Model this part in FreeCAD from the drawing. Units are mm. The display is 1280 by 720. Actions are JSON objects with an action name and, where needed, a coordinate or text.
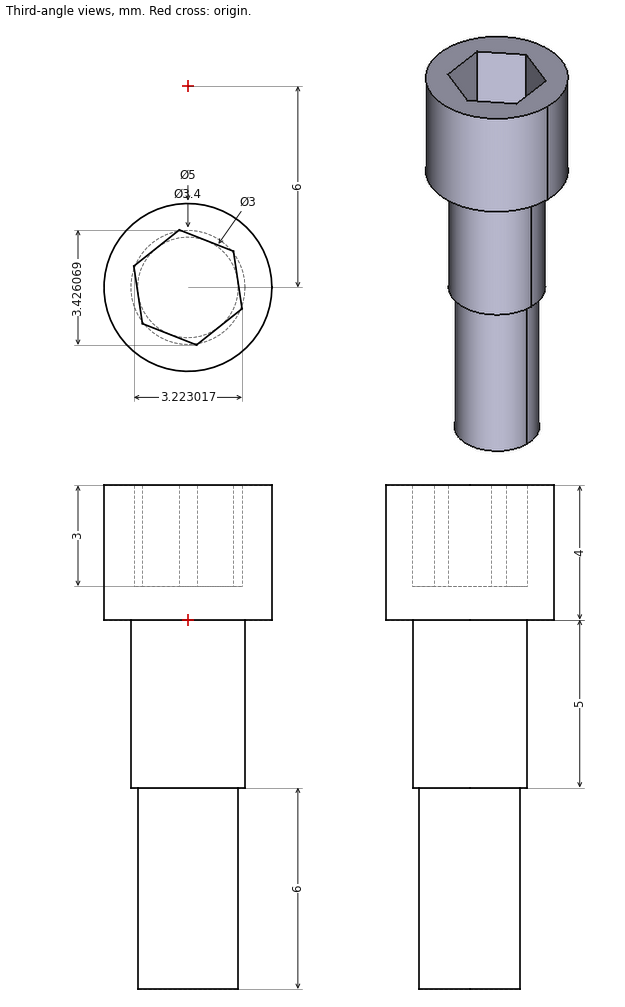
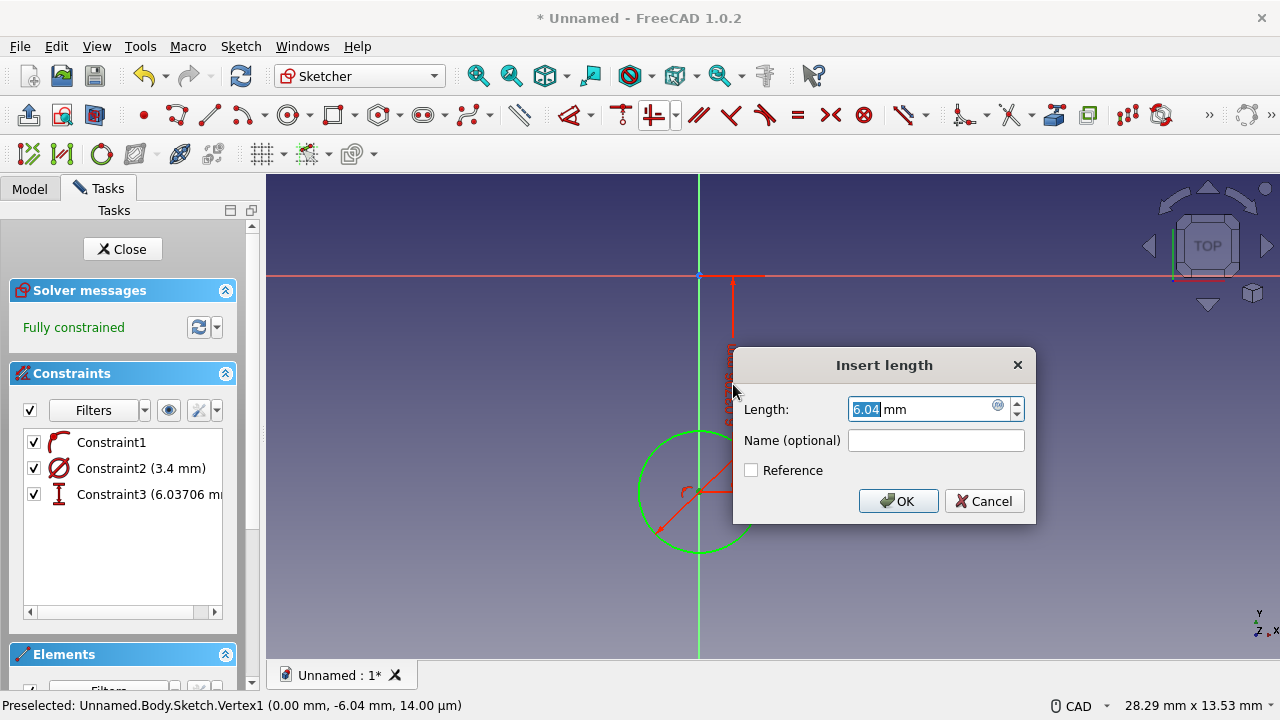
{"action": "type", "text": "6"}
{"action": "key", "text": "Return"}
{"action": "key", "text": "Escape"}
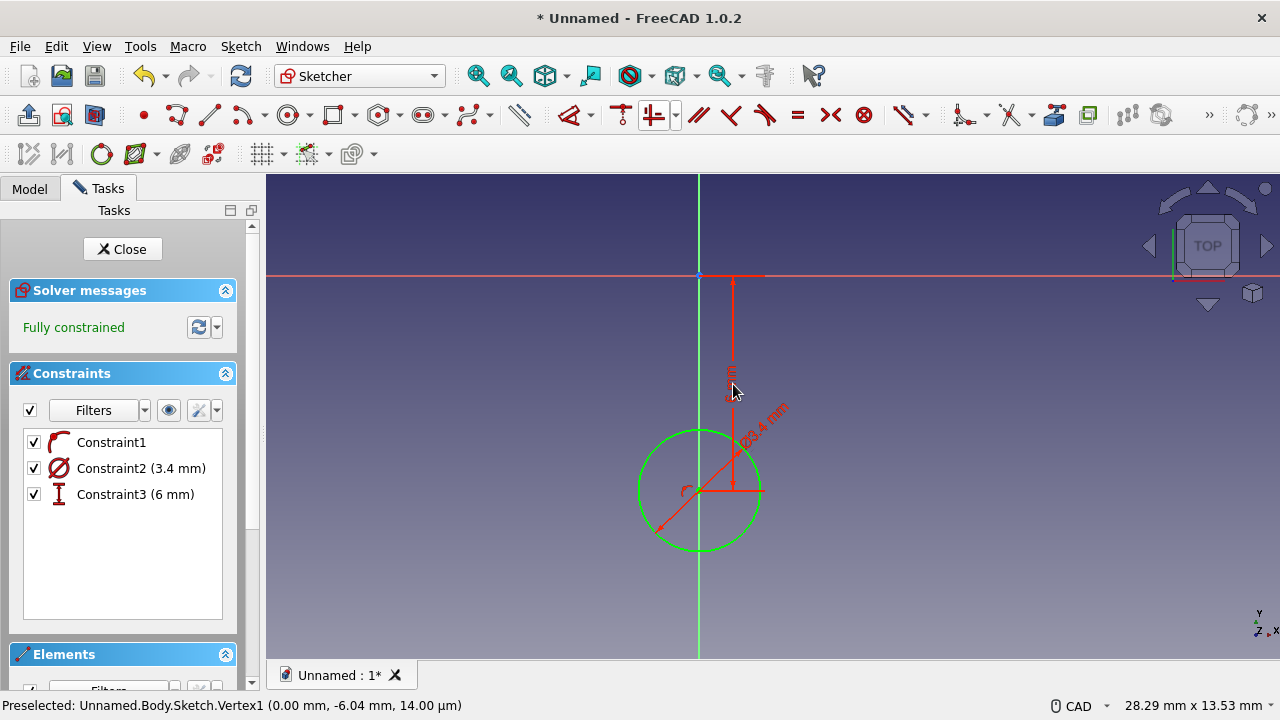
{"action": "left_click", "coordinate": [123, 249]}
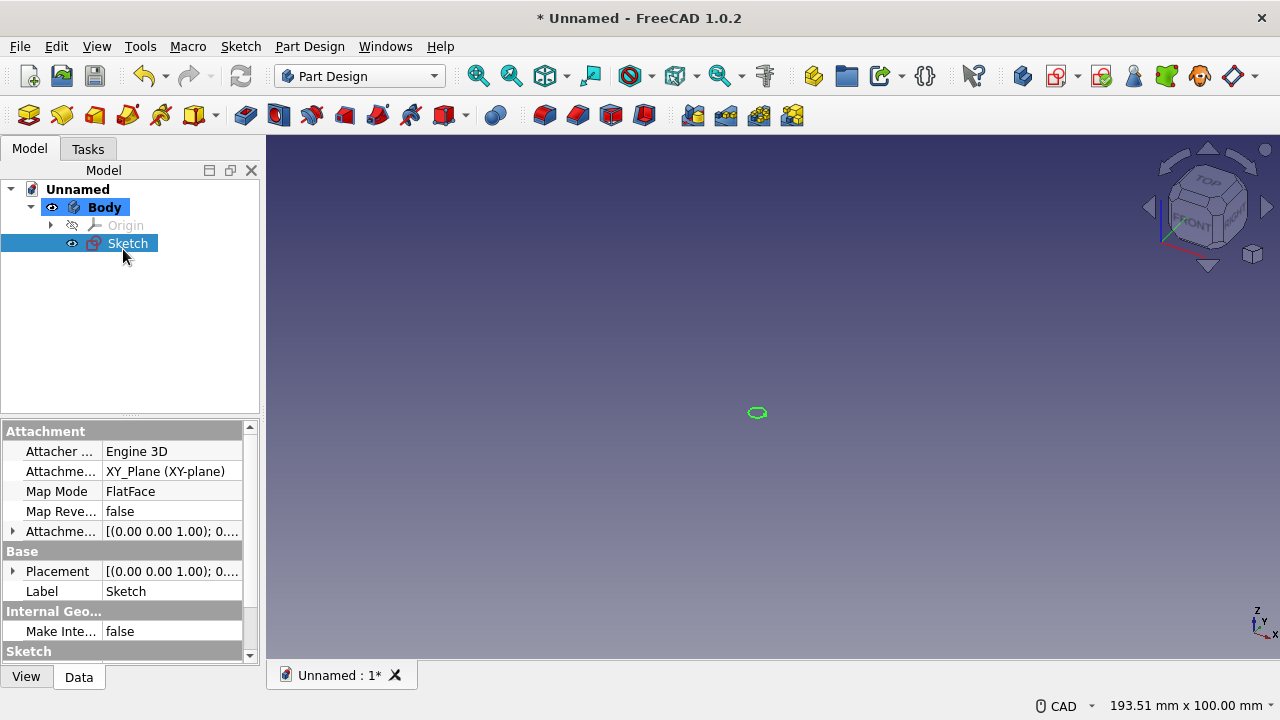
{"action": "left_click", "coordinate": [29, 116]}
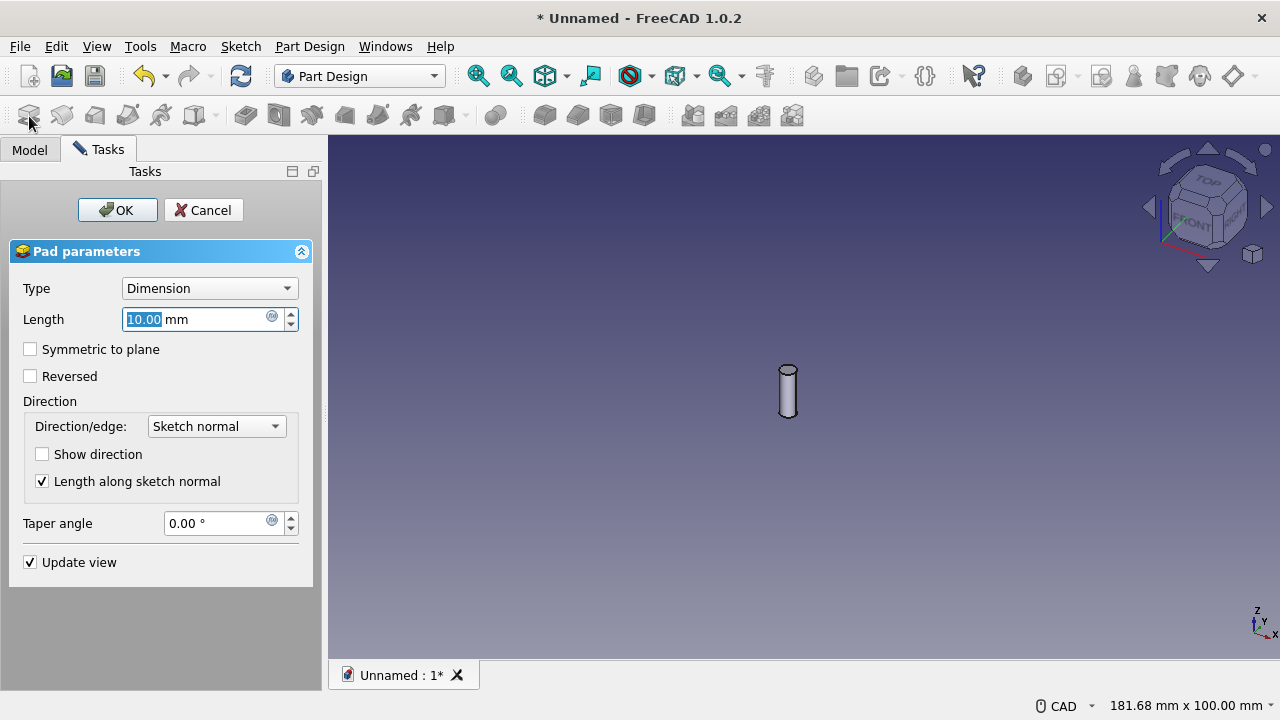
{"action": "type", "text": "5"}
{"action": "key", "text": "Tab"}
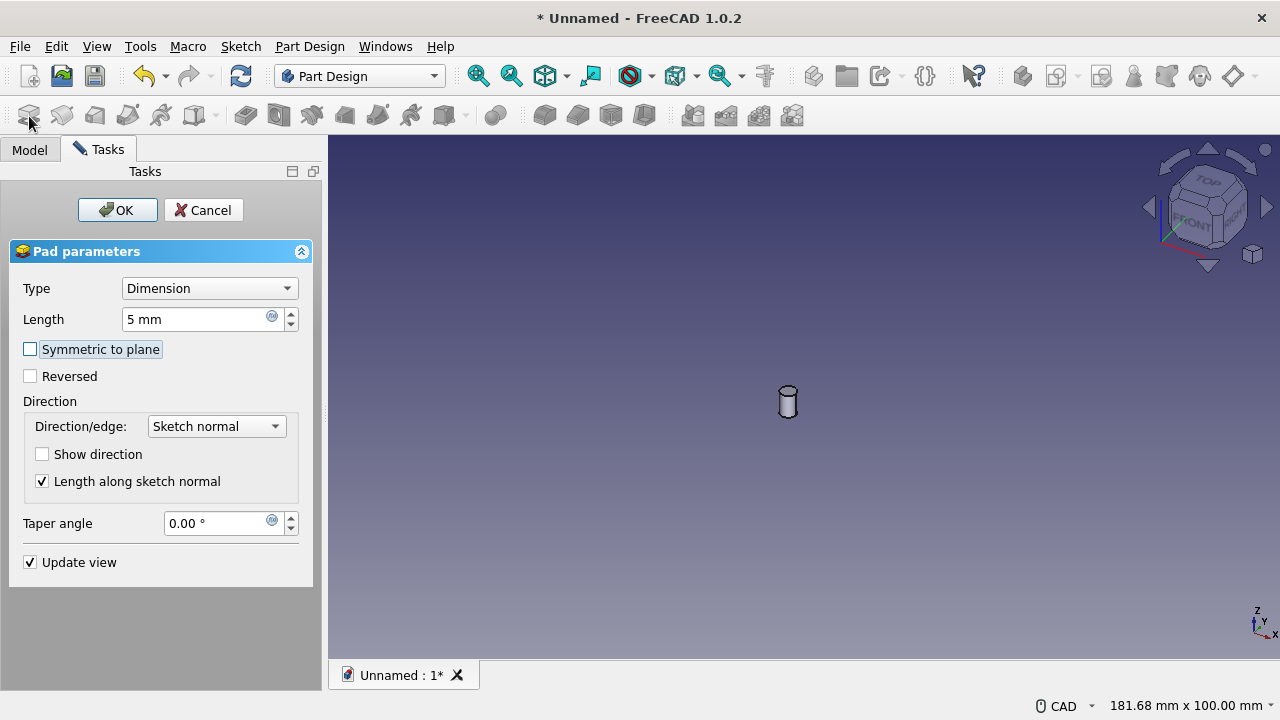
{"action": "left_click", "coordinate": [31, 376]}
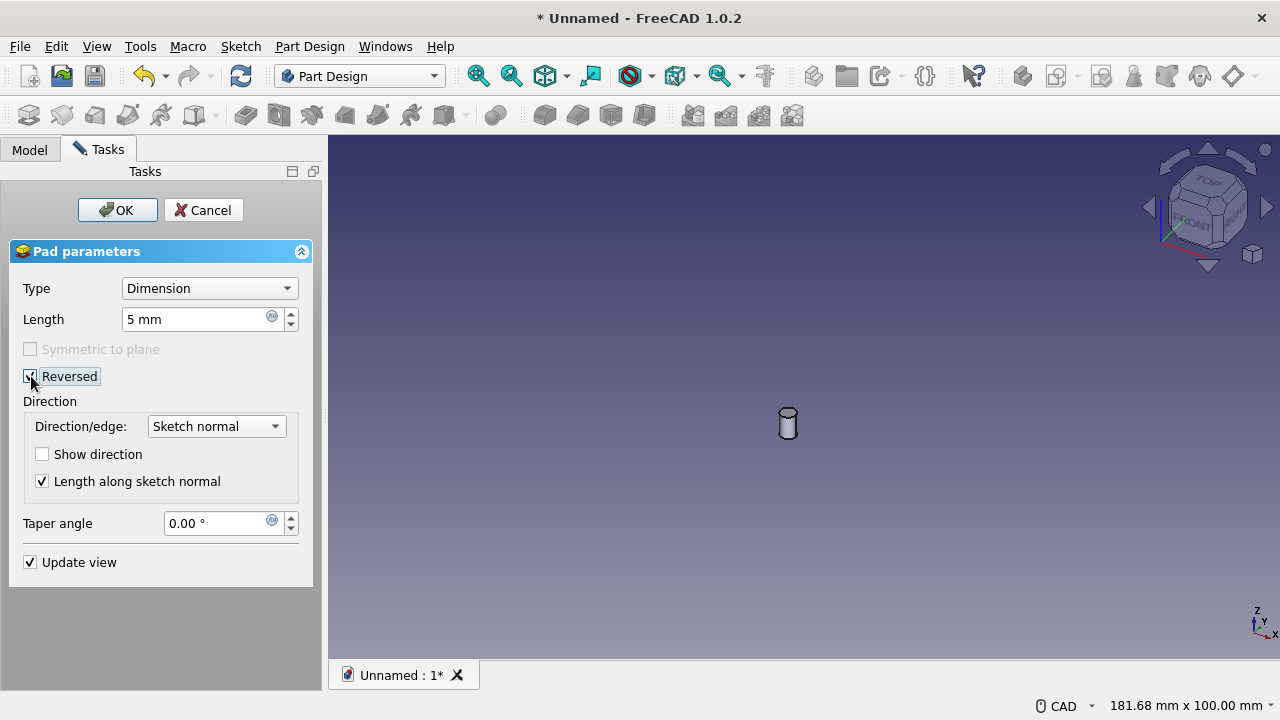
{"action": "left_click", "coordinate": [118, 210]}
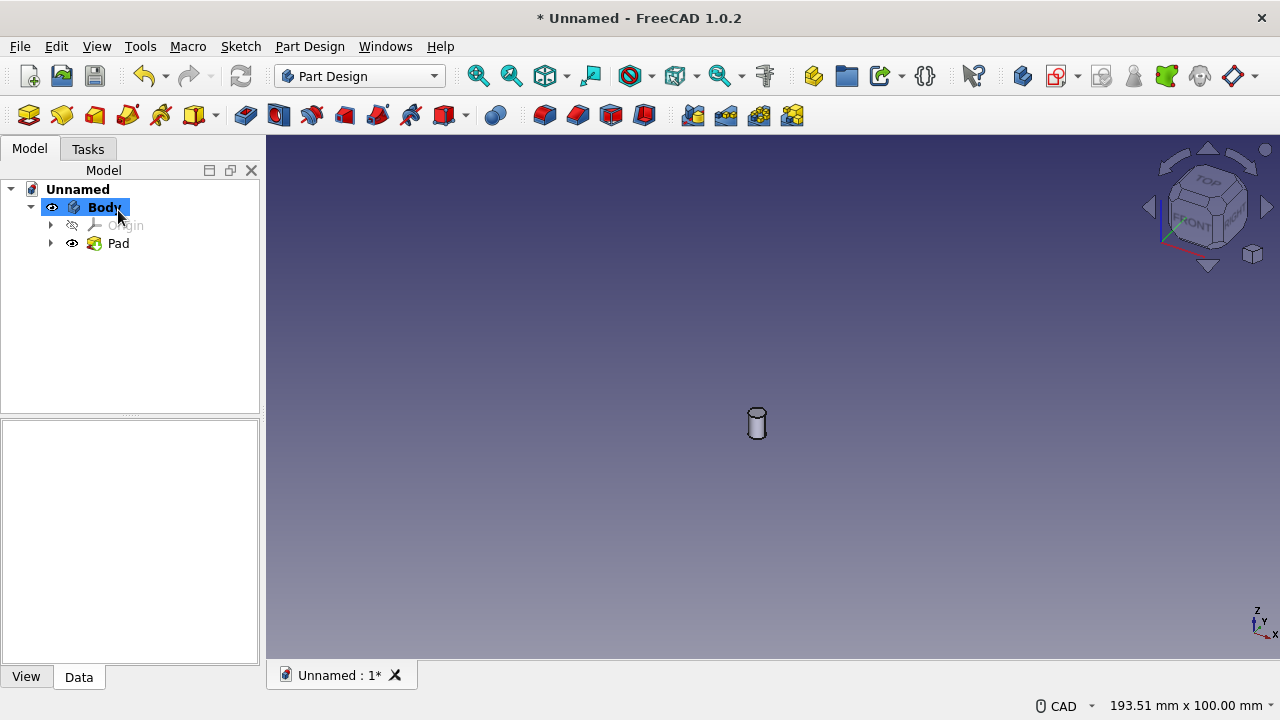
{"action": "left_click", "coordinate": [479, 76]}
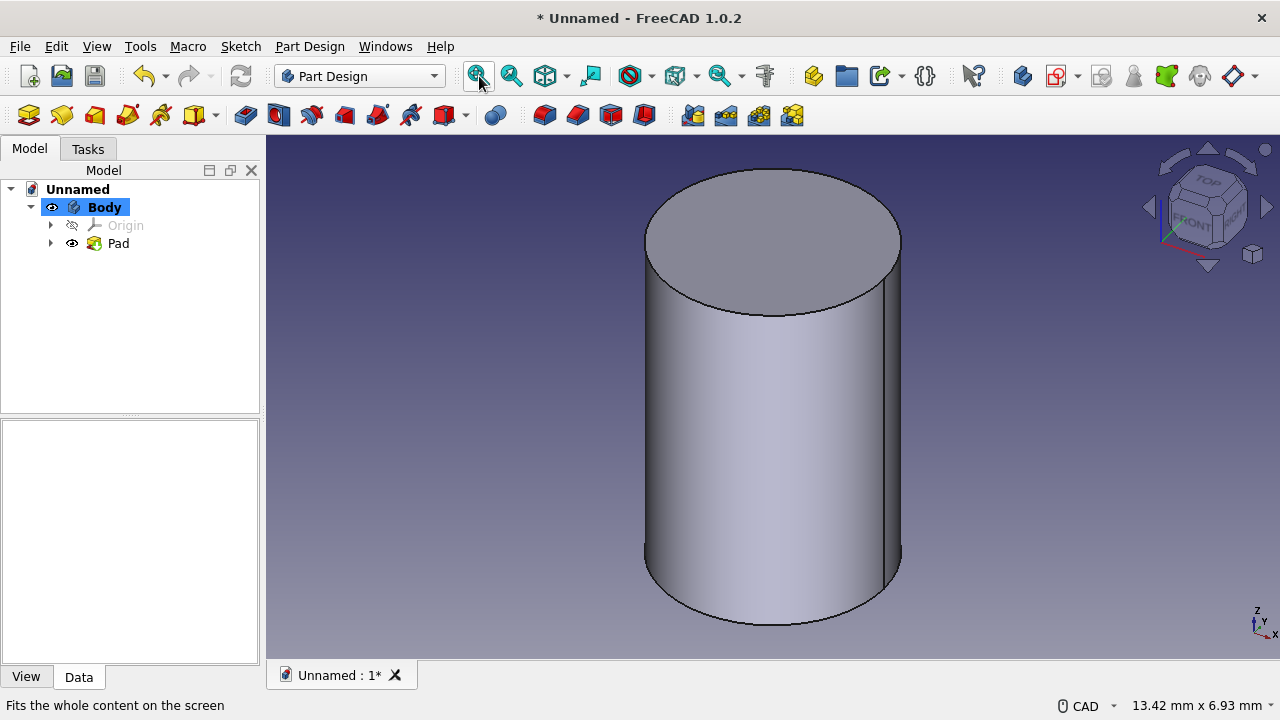
{"action": "key", "text": "5"}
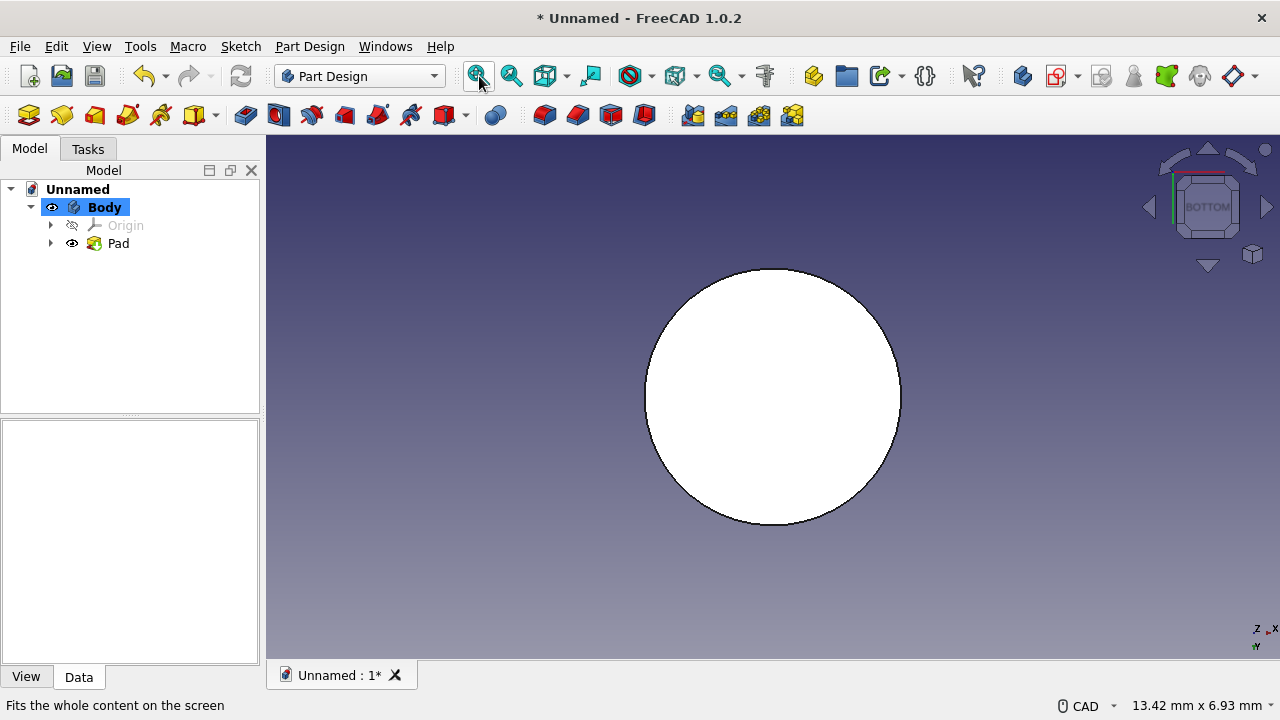
{"action": "left_click", "coordinate": [773, 396]}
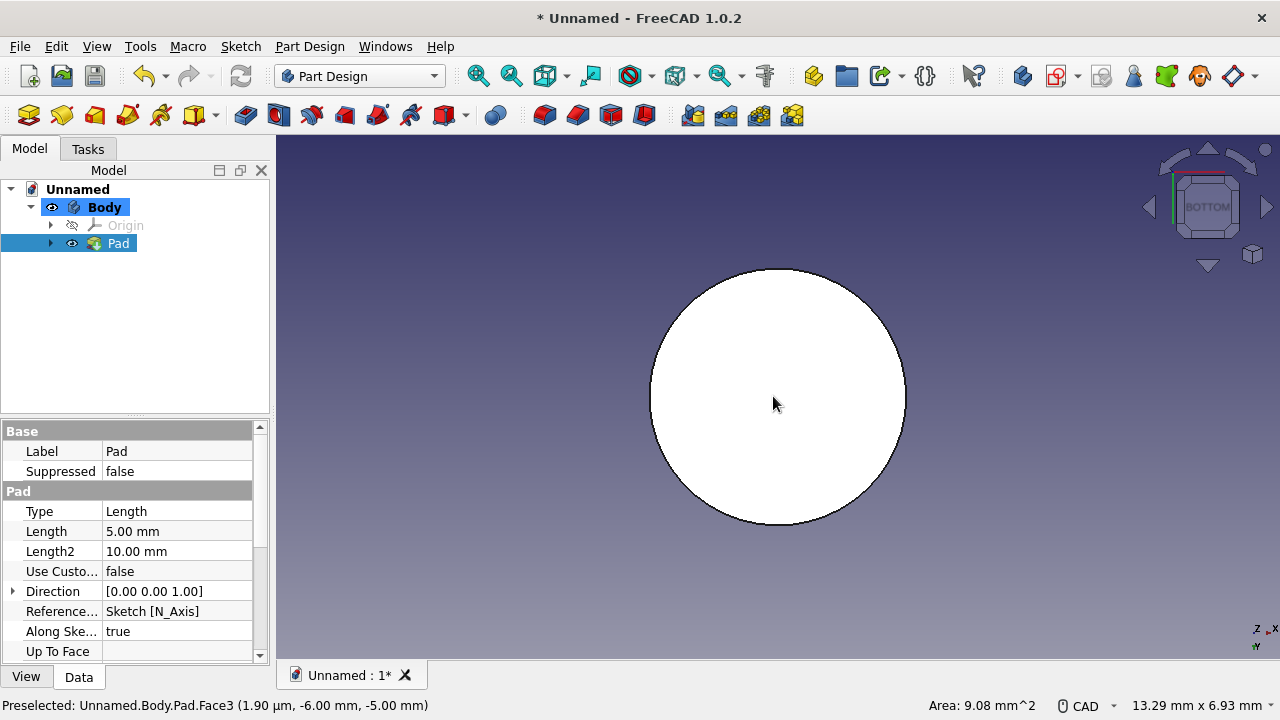
{"action": "left_click", "coordinate": [1056, 76]}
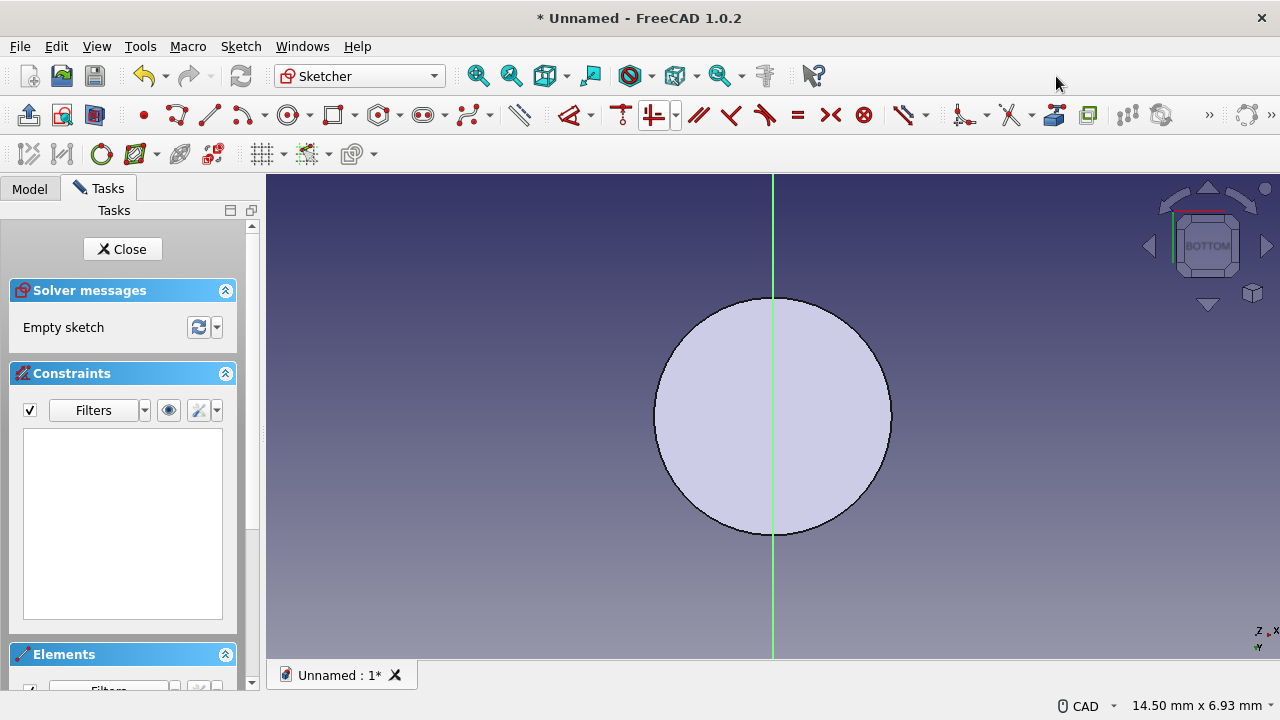
{"action": "scroll", "coordinate": [912, 416], "scroll_direction": "up", "scroll_amount": 2}